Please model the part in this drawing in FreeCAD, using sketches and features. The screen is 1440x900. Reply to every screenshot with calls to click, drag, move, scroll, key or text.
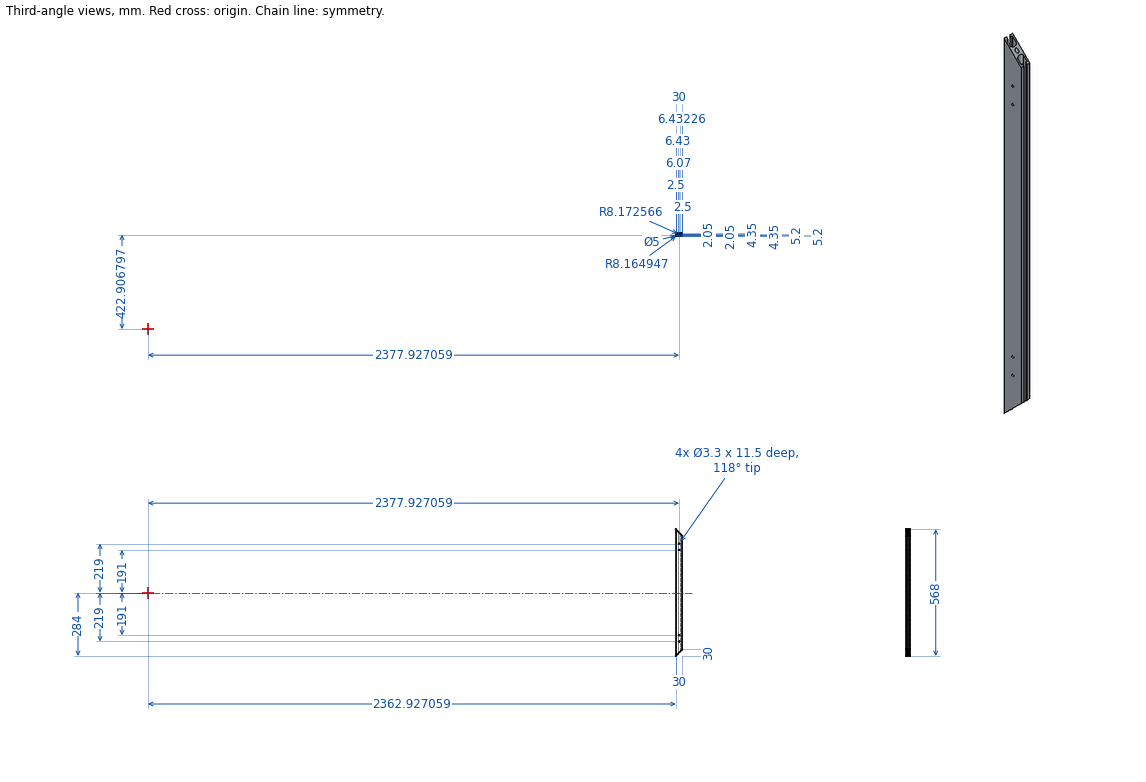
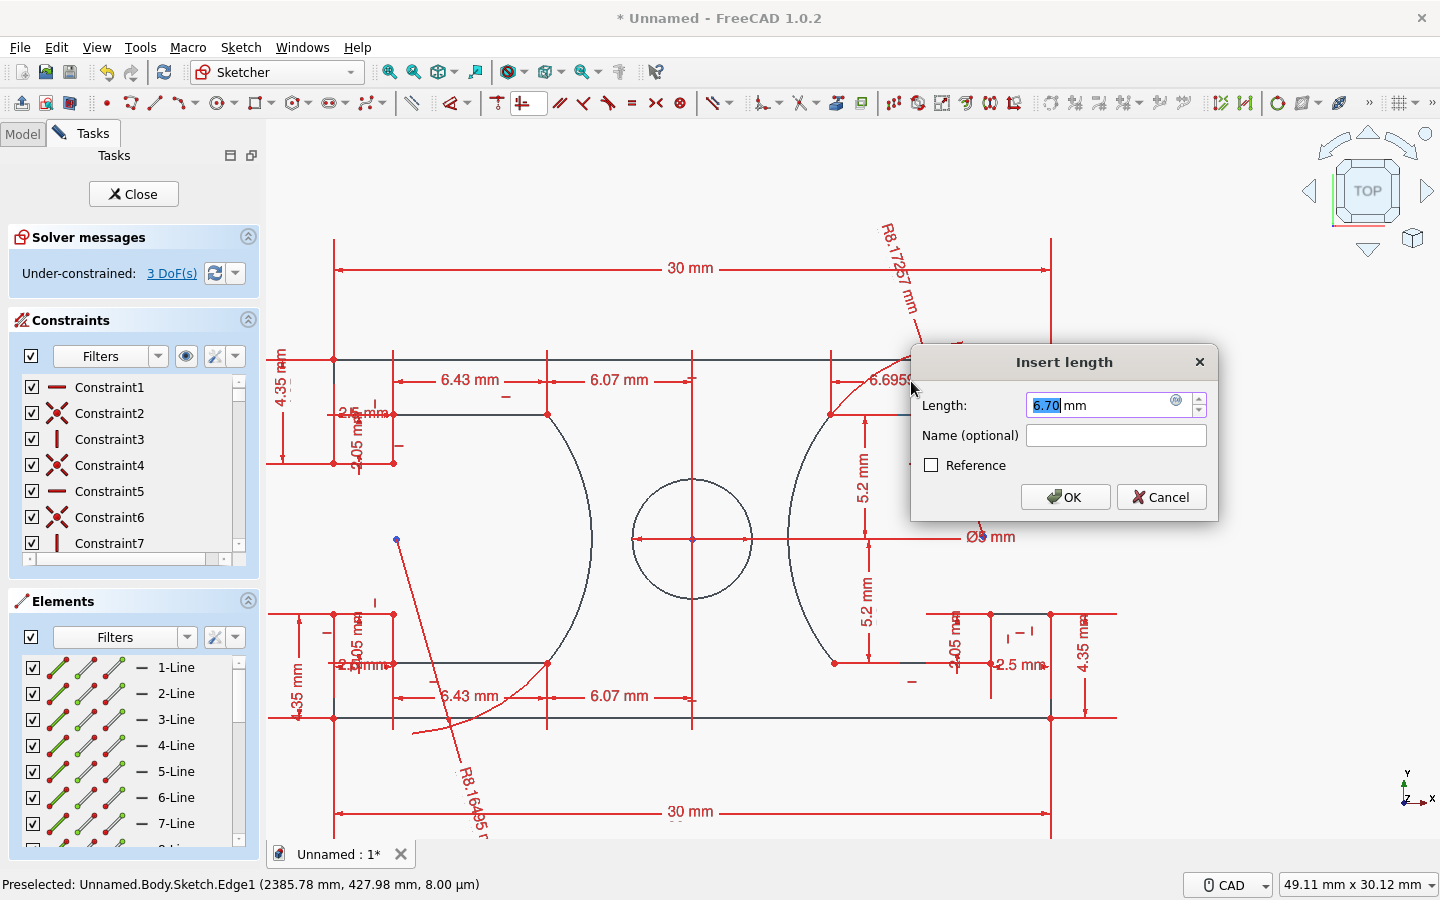
text(6.43226)
key(Return)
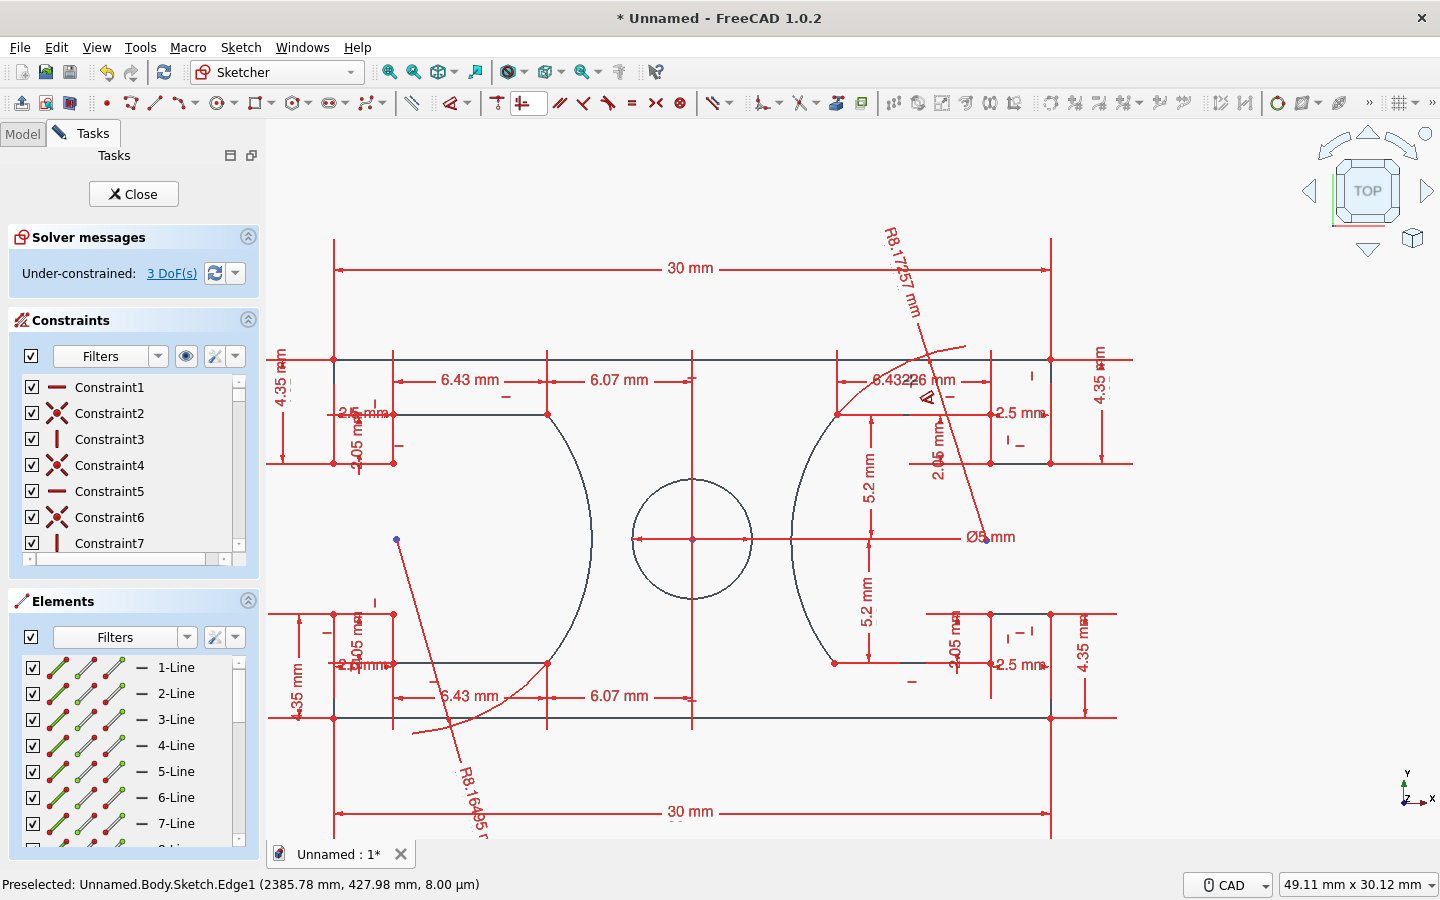
click(944, 663)
click(913, 697)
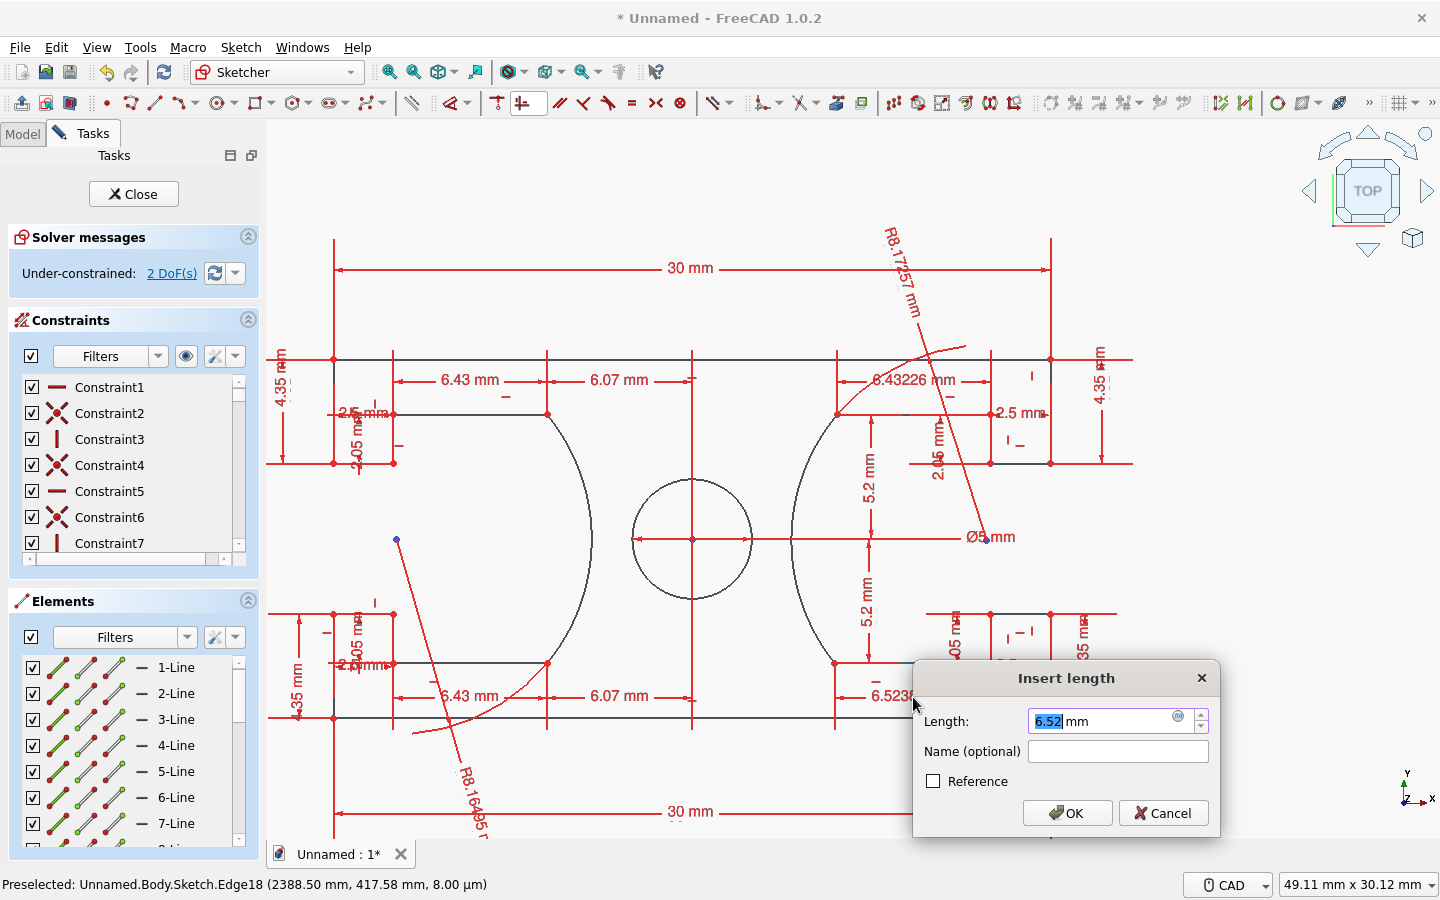
text(6.43226)
key(Return)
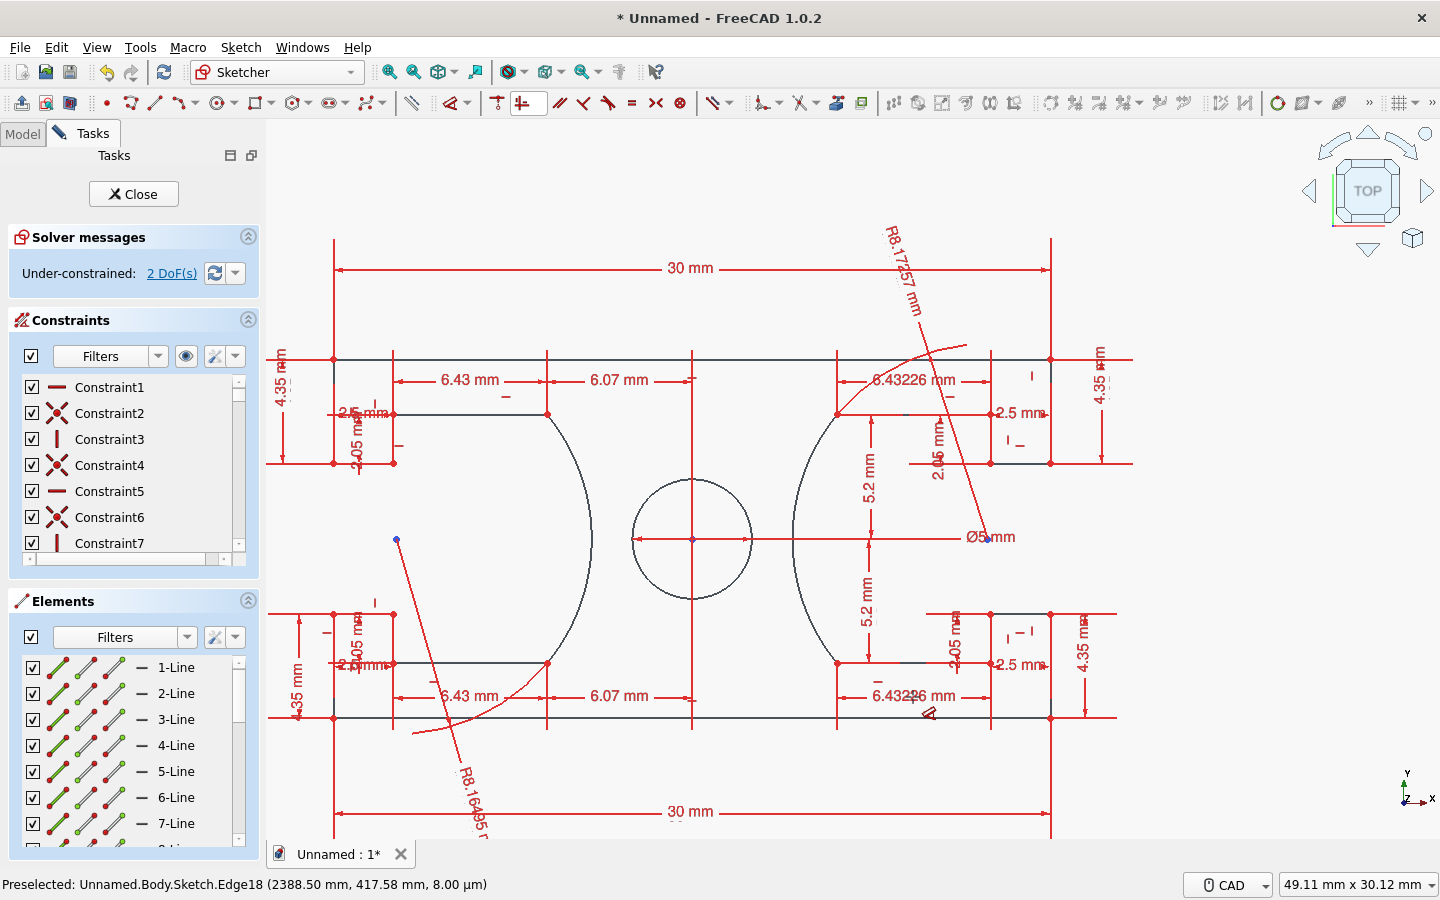
click(692, 539)
click(726, 675)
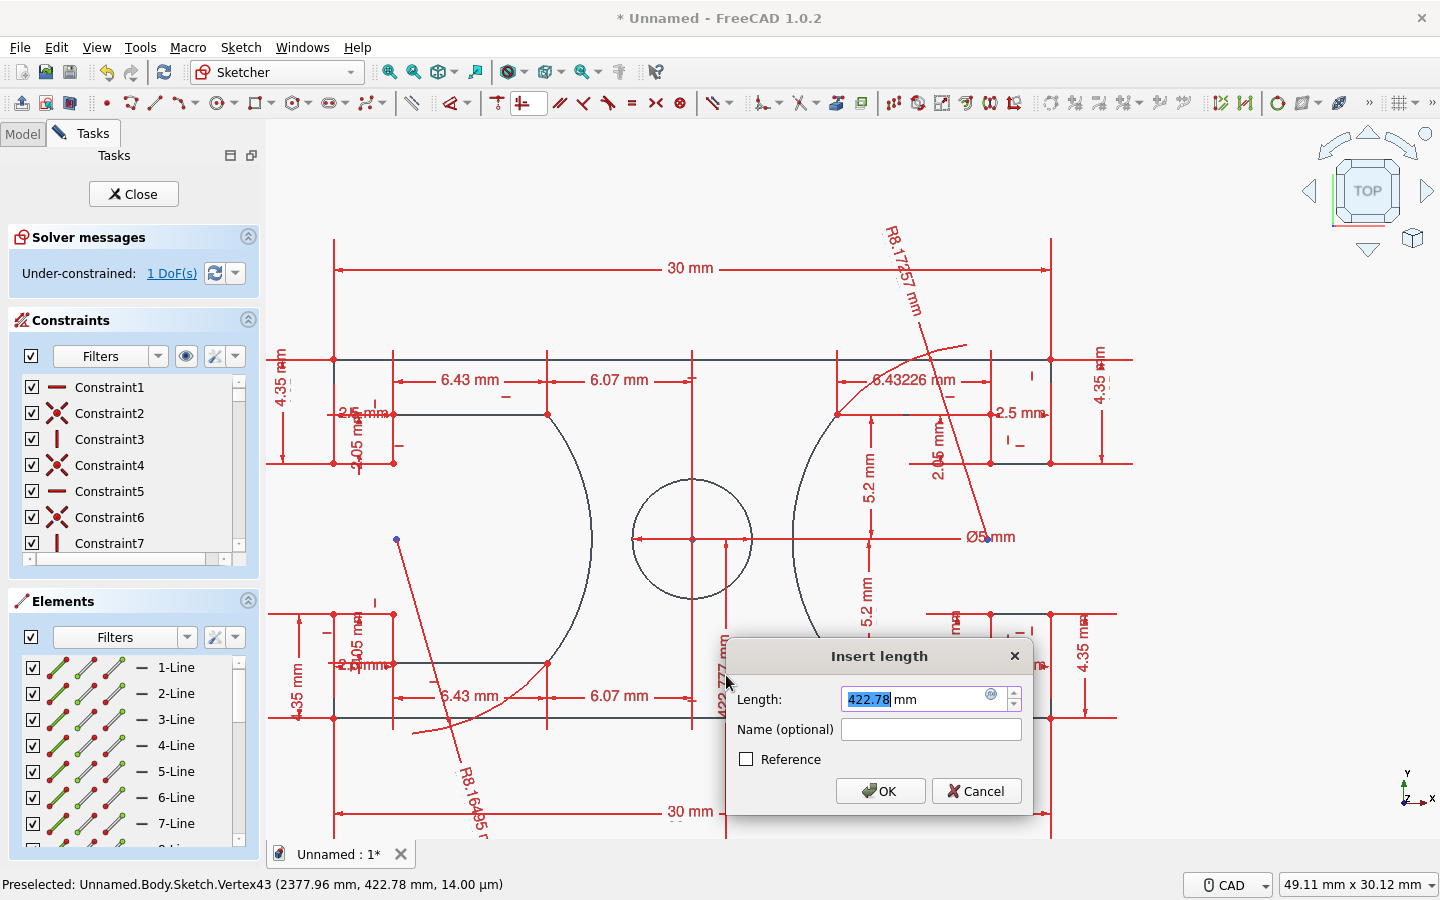
text(422.906797)
key(Return)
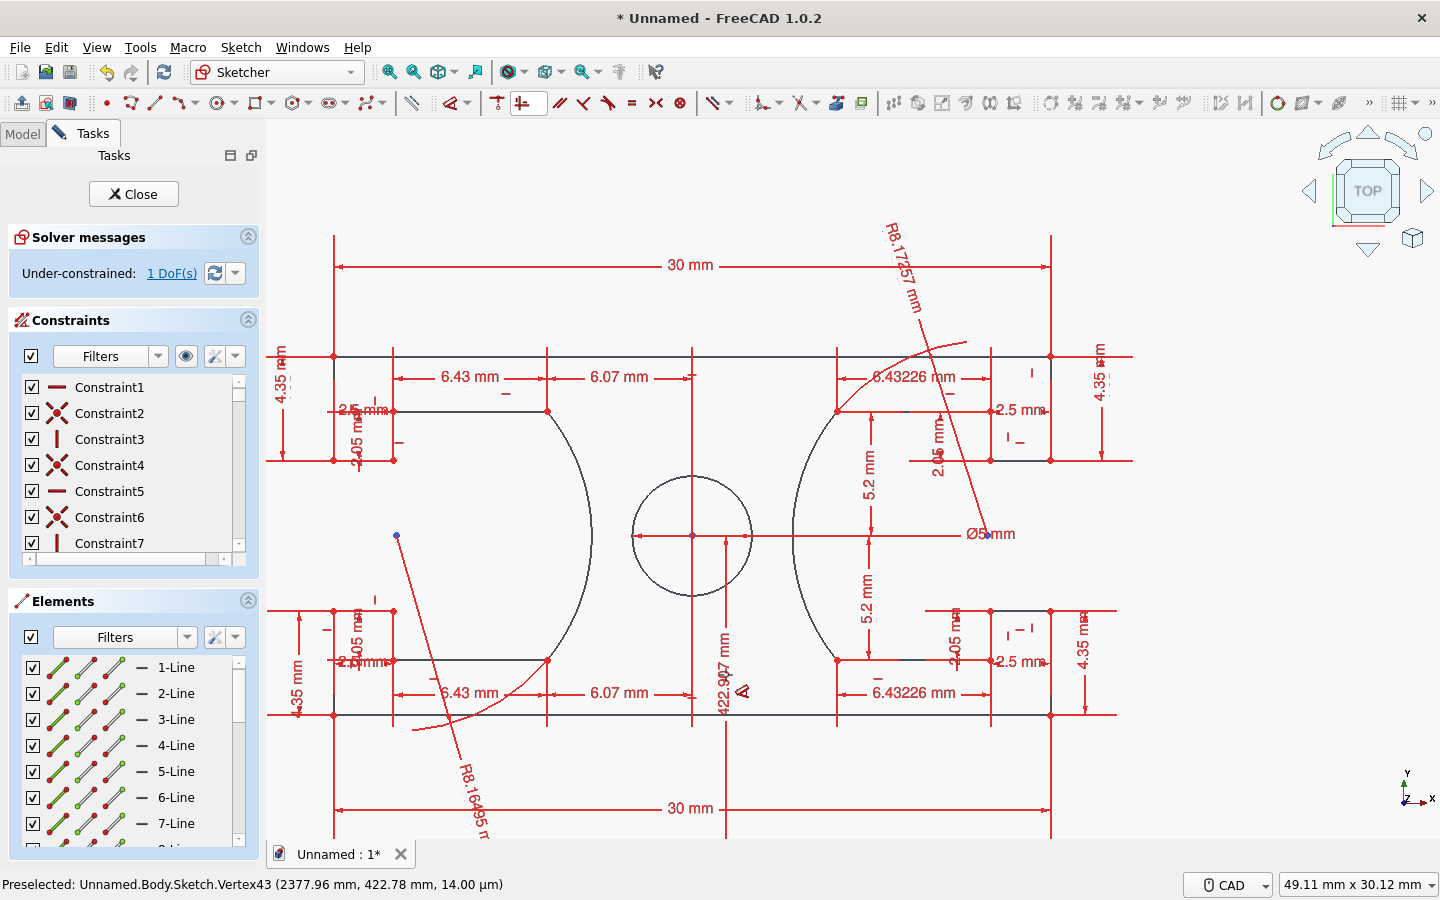
click(692, 536)
click(493, 502)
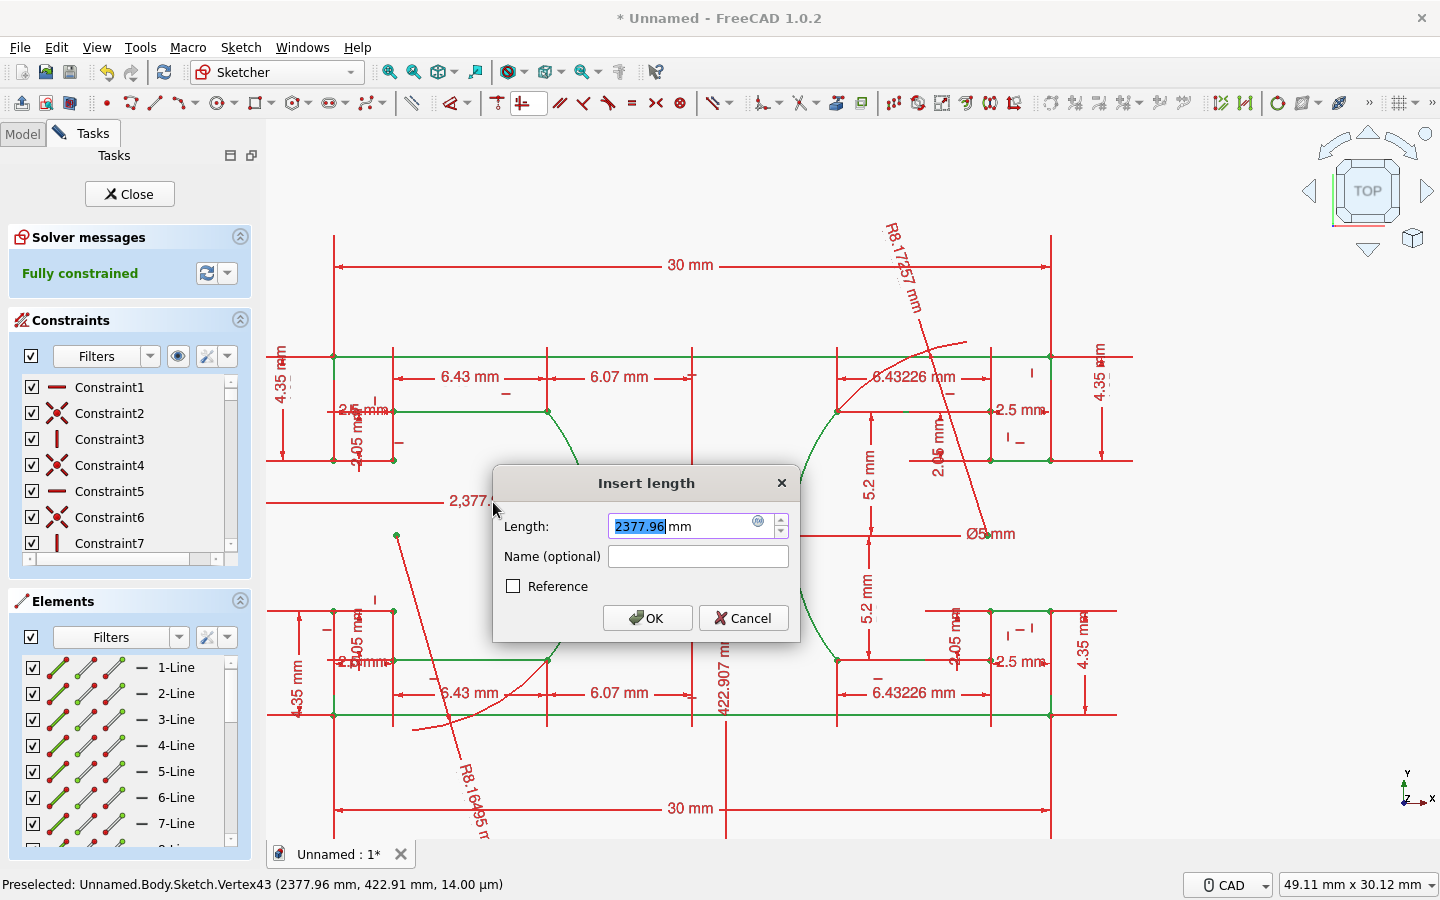
text(2377.927059)
key(Return)
key(Escape)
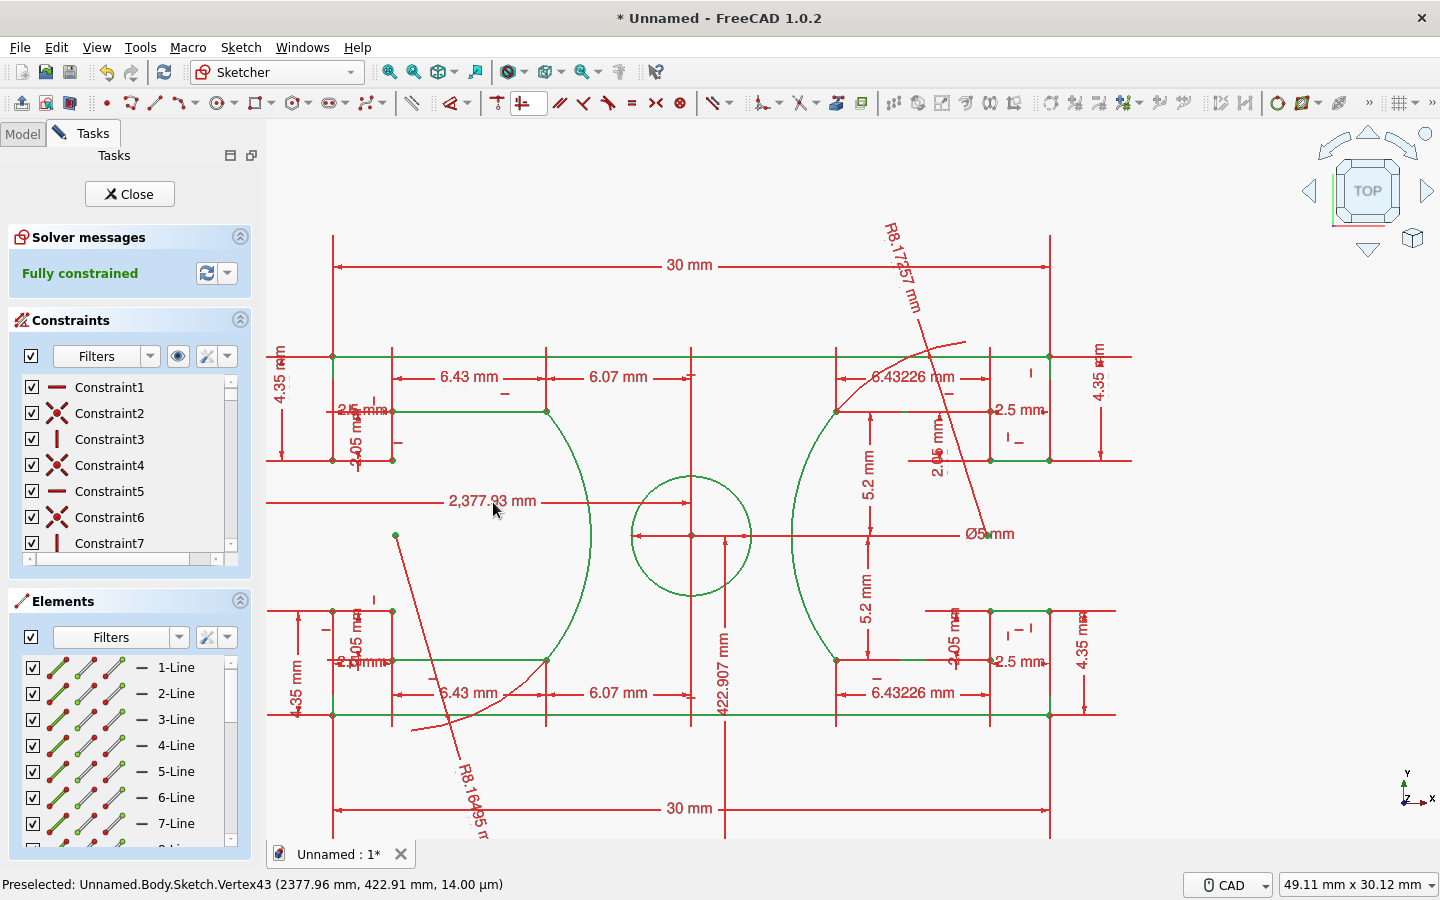
click(130, 194)